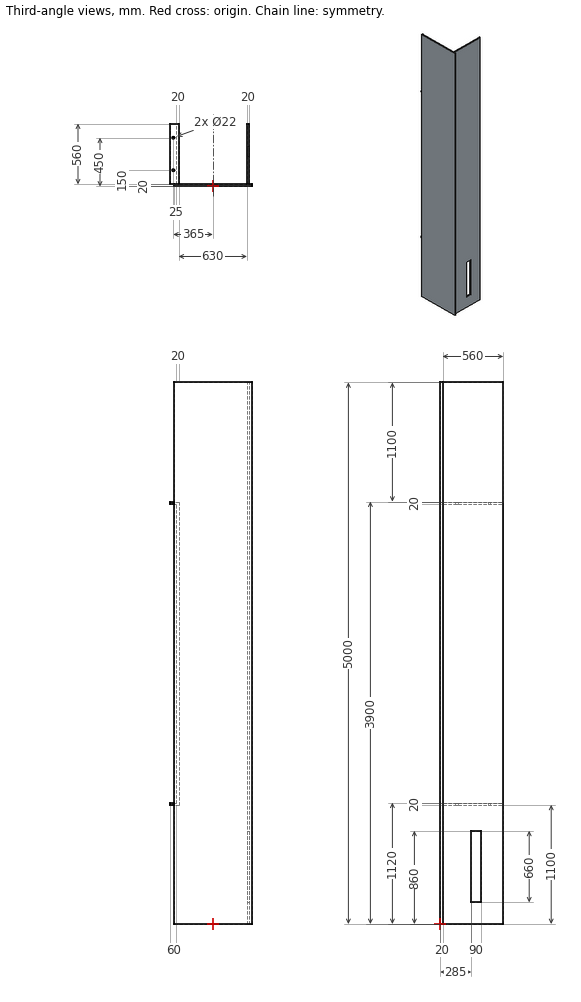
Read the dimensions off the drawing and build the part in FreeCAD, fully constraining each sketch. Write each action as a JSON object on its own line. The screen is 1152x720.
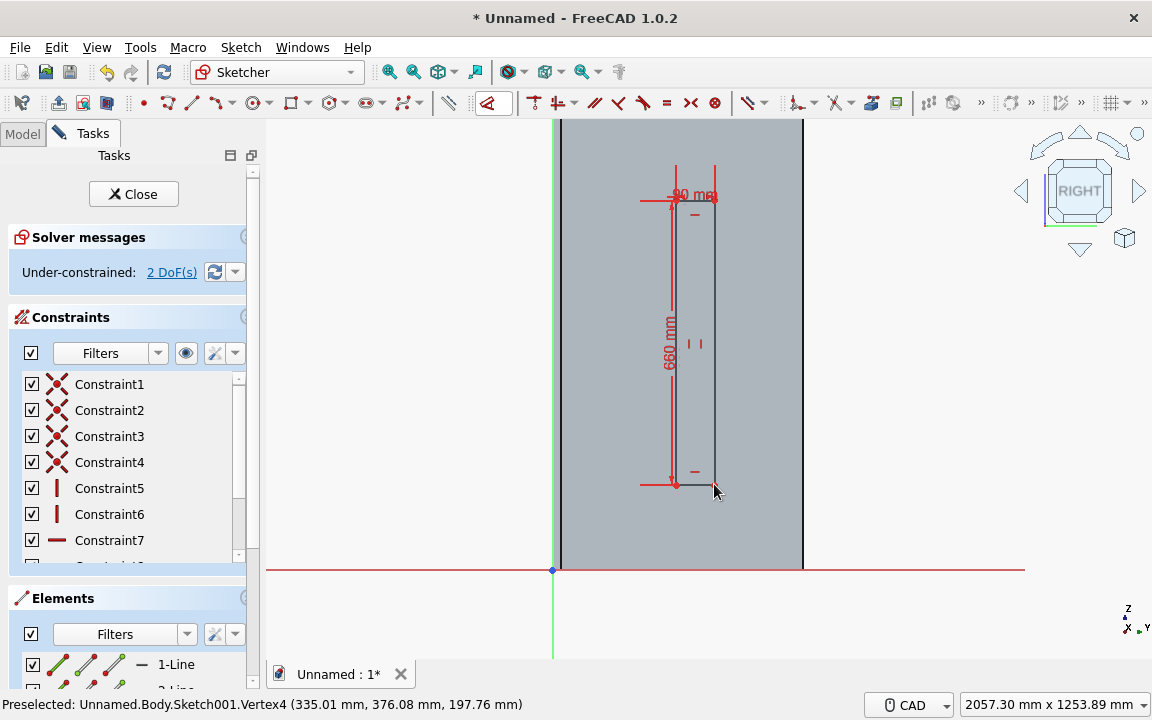
{"action": "left_click", "coordinate": [676, 201]}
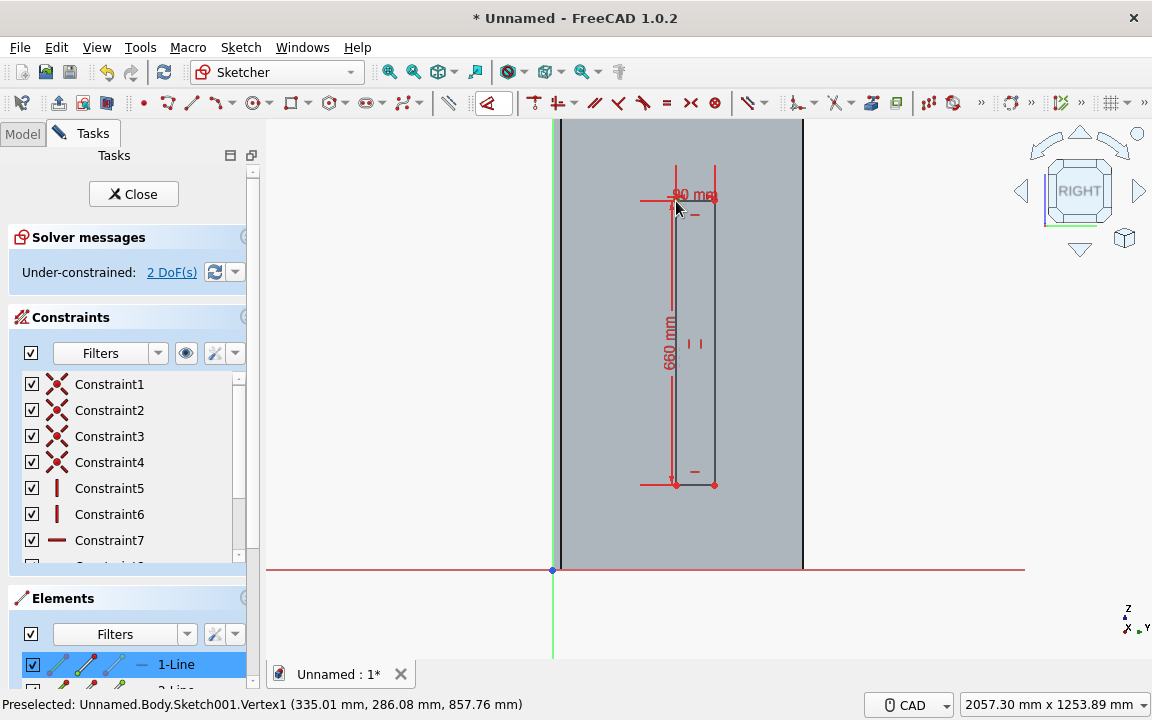
{"action": "left_click", "coordinate": [506, 104]}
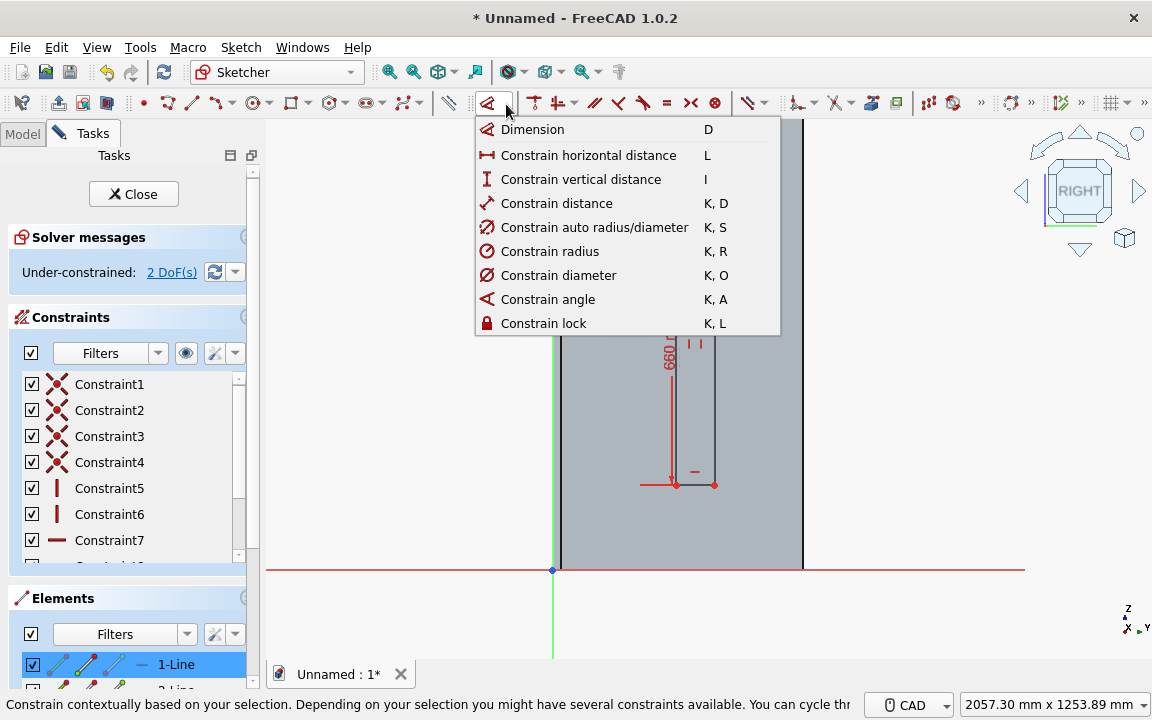
{"action": "left_click", "coordinate": [628, 155]}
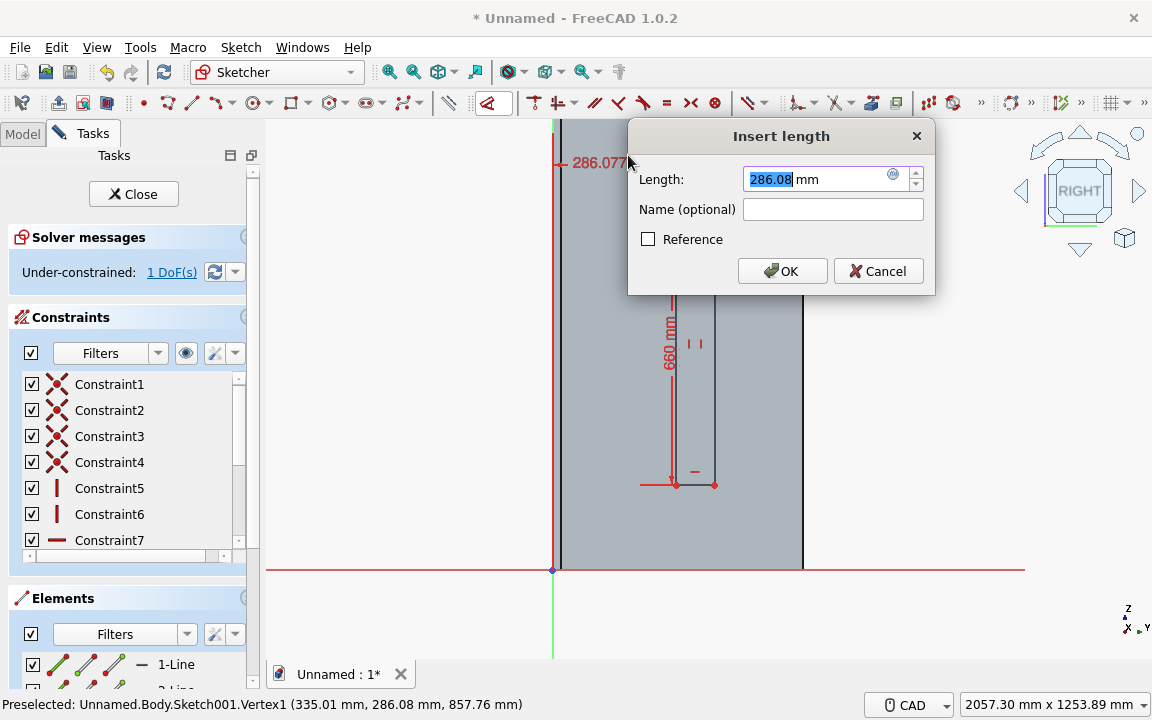
{"action": "type", "text": "285"}
{"action": "key", "text": "Return"}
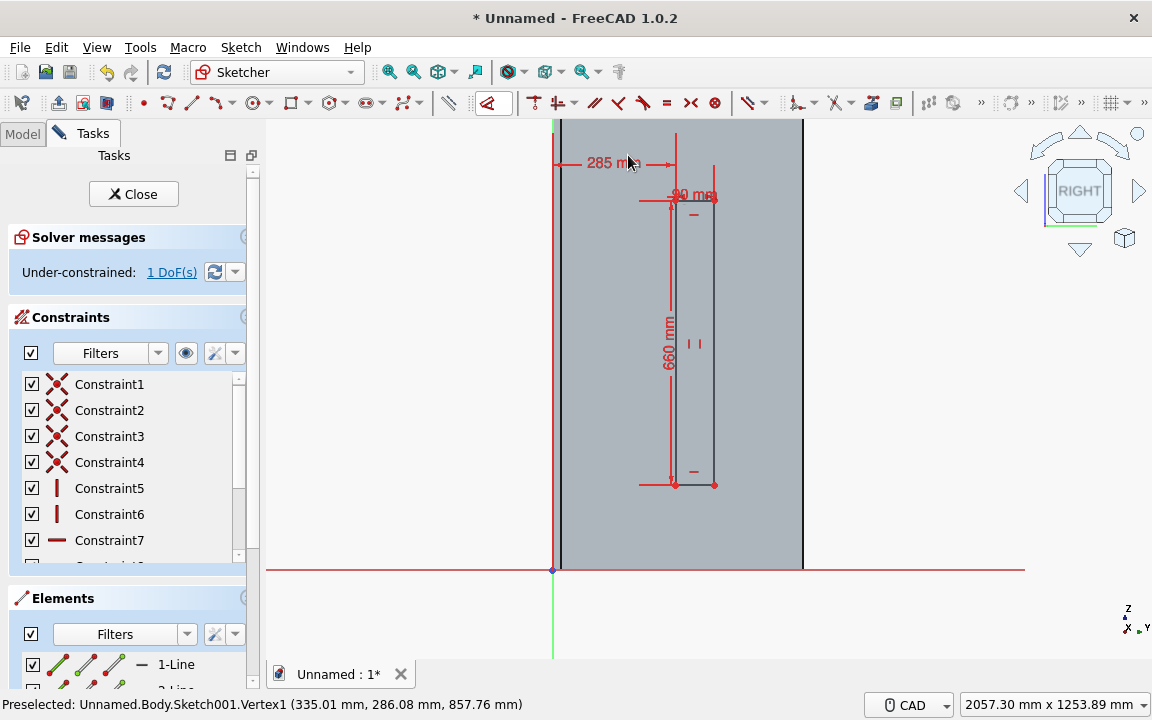
{"action": "left_click", "coordinate": [676, 201]}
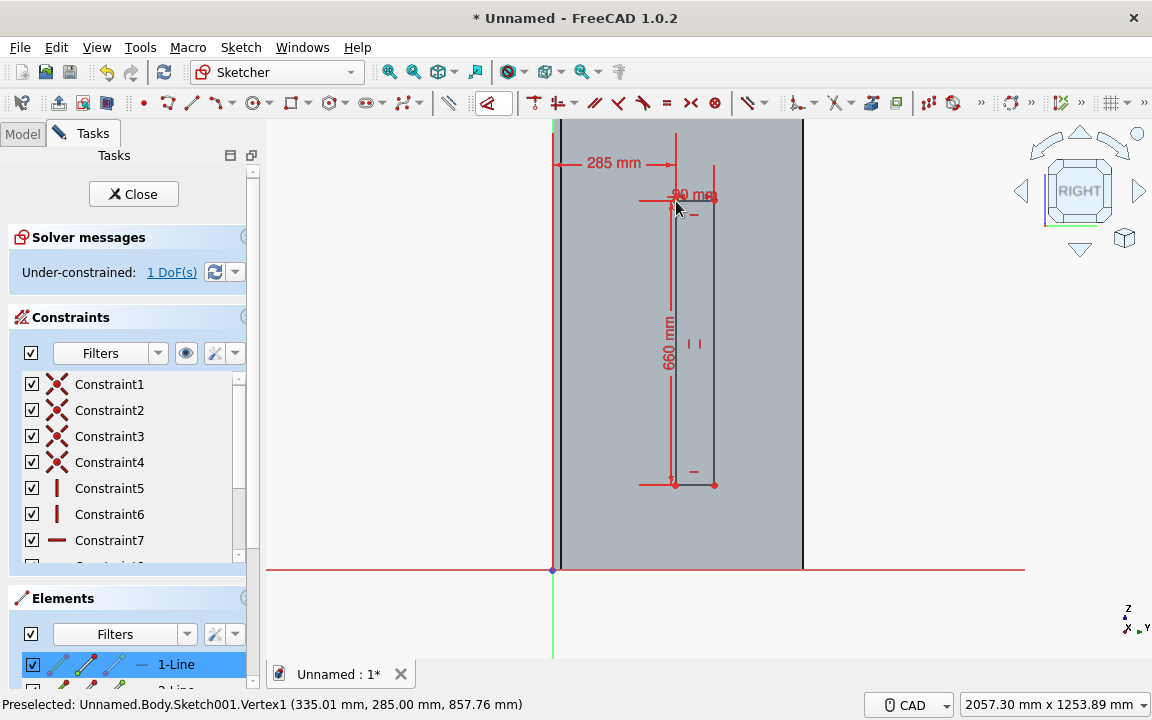
{"action": "left_click", "coordinate": [506, 104]}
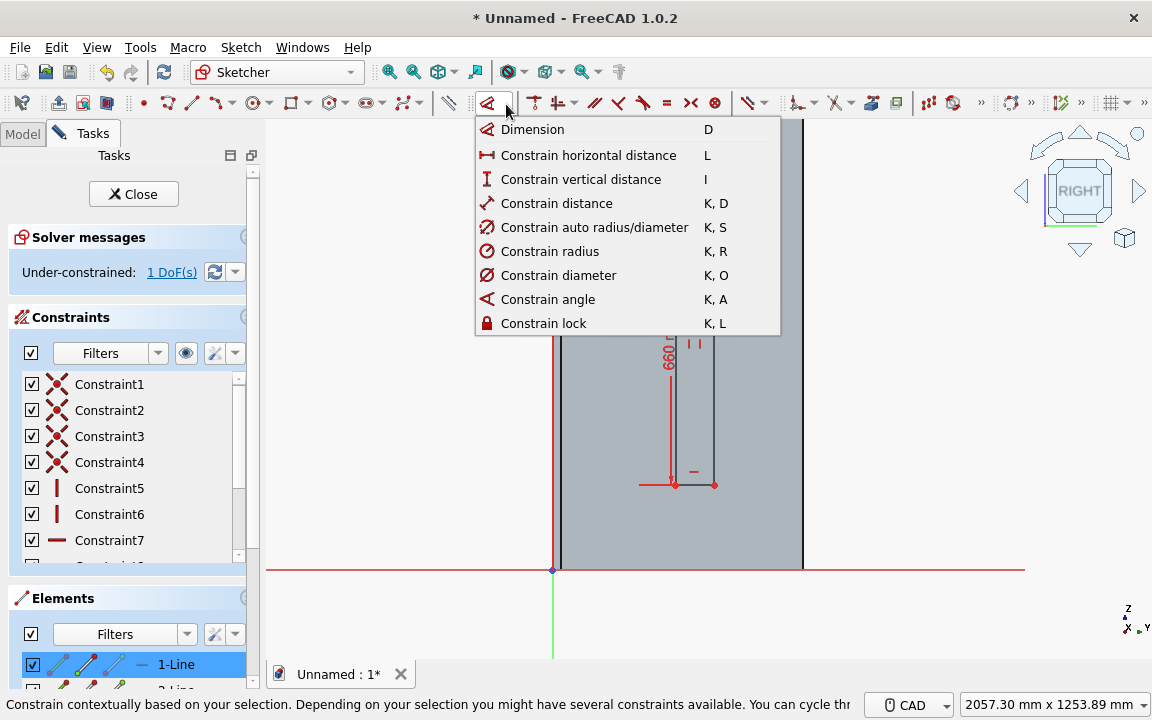
{"action": "left_click", "coordinate": [628, 179]}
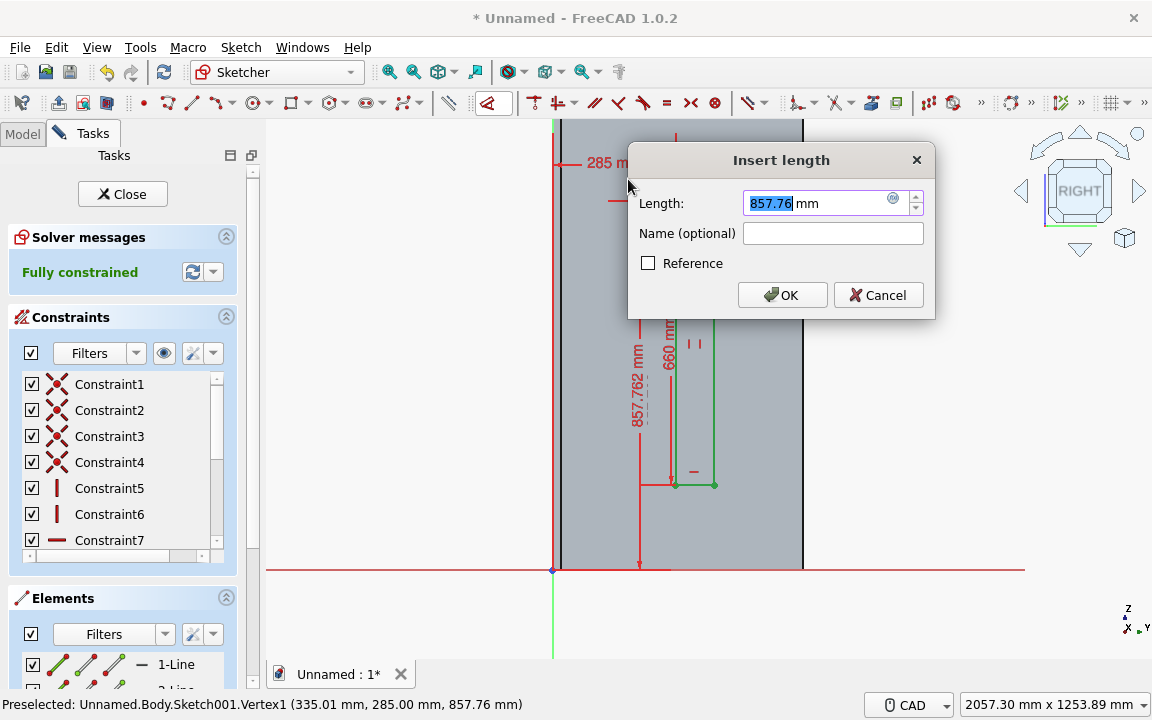
{"action": "type", "text": "860"}
{"action": "key", "text": "Return"}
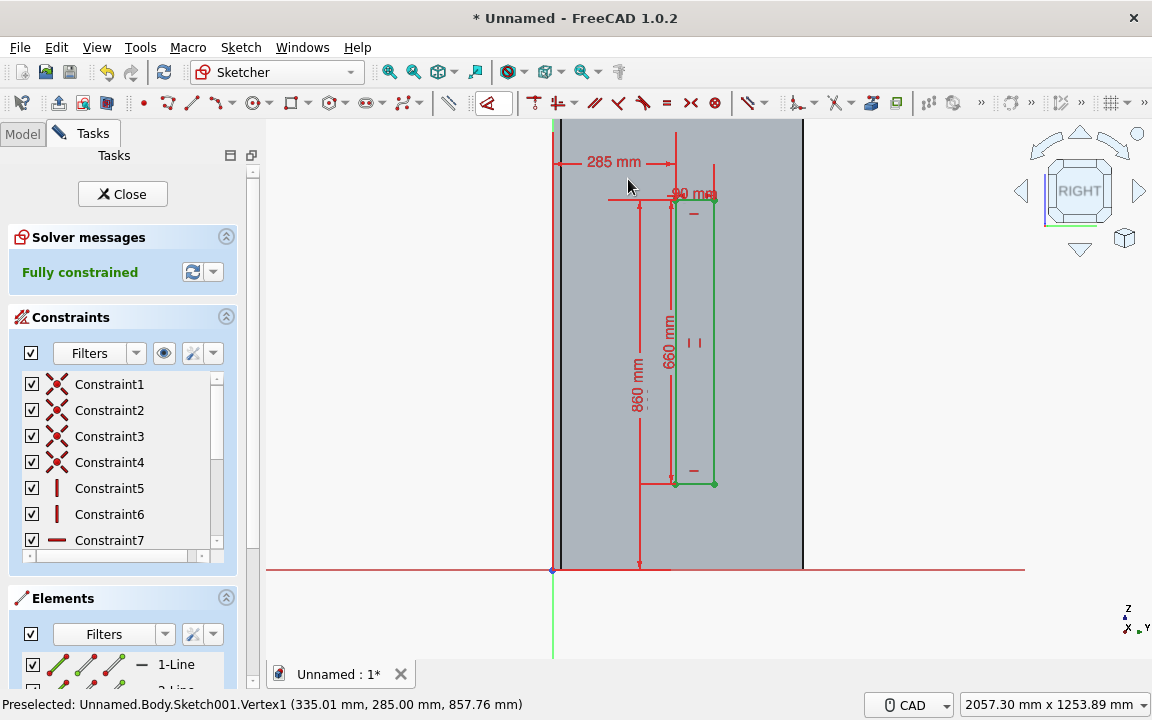
{"action": "left_click", "coordinate": [123, 194]}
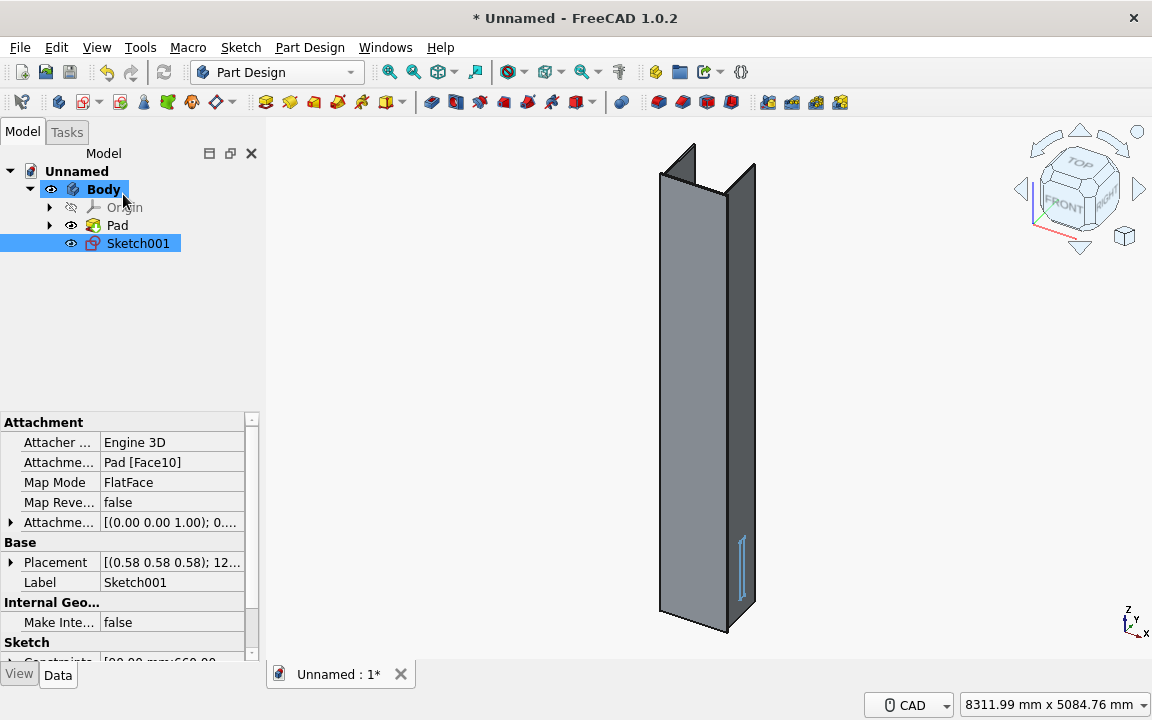
{"action": "left_click", "coordinate": [432, 102]}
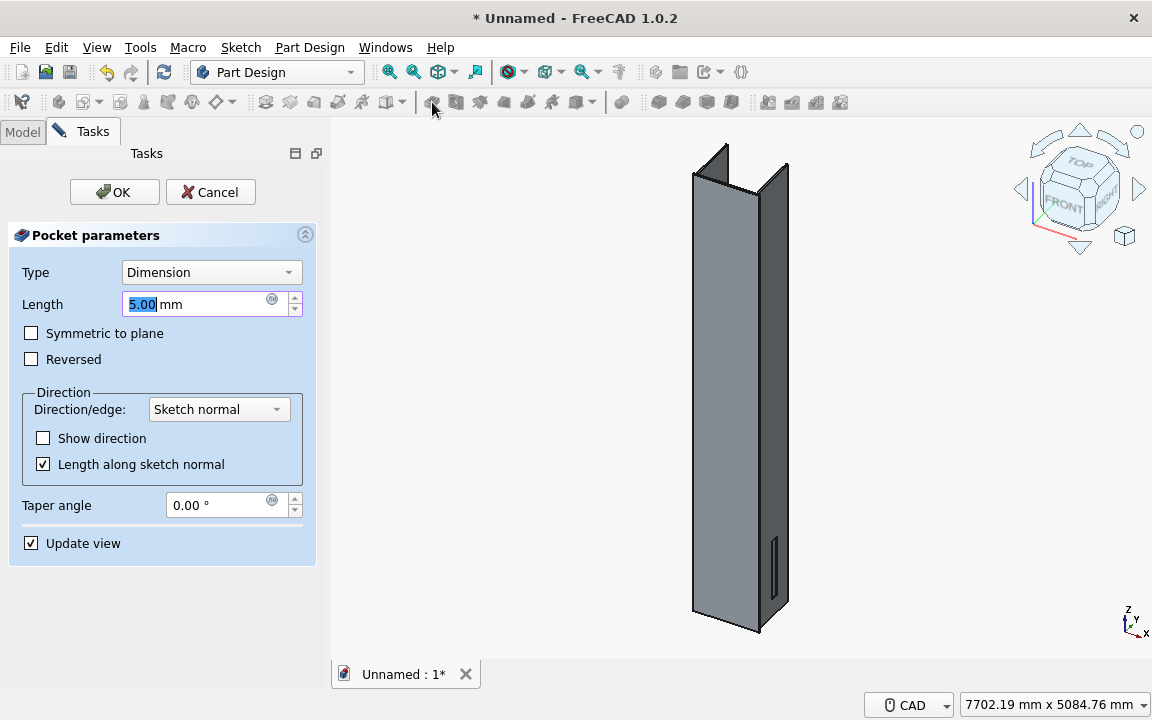
{"action": "left_click", "coordinate": [212, 272]}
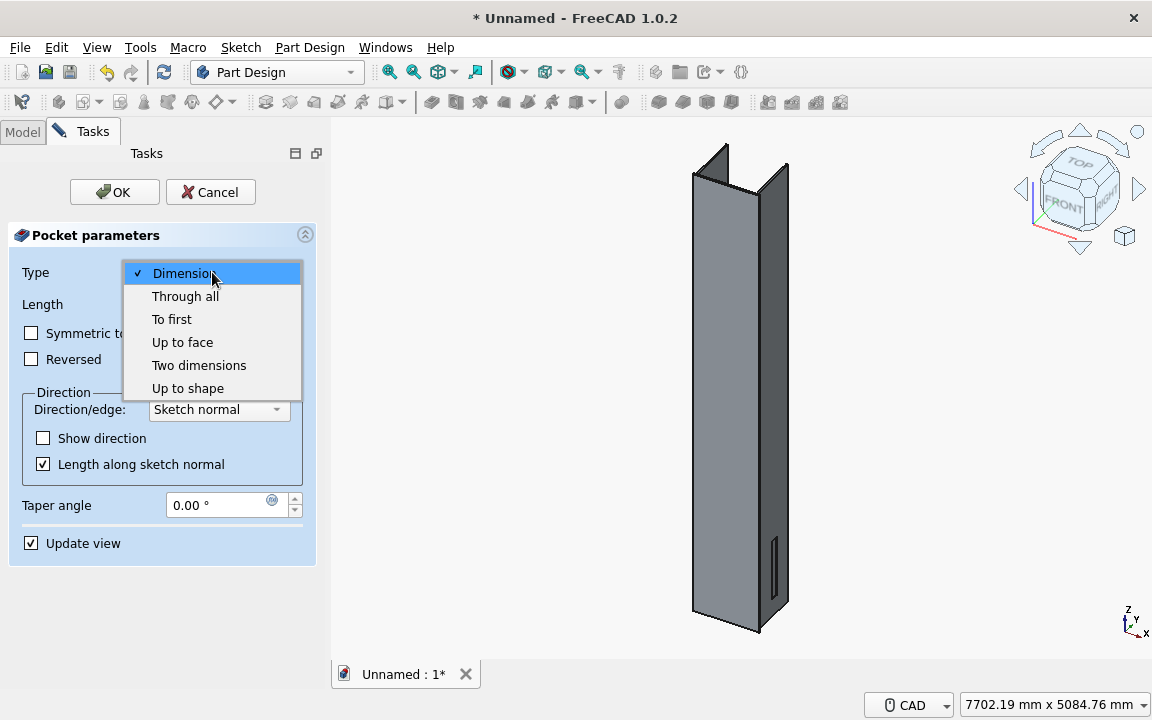
{"action": "left_click", "coordinate": [212, 320]}